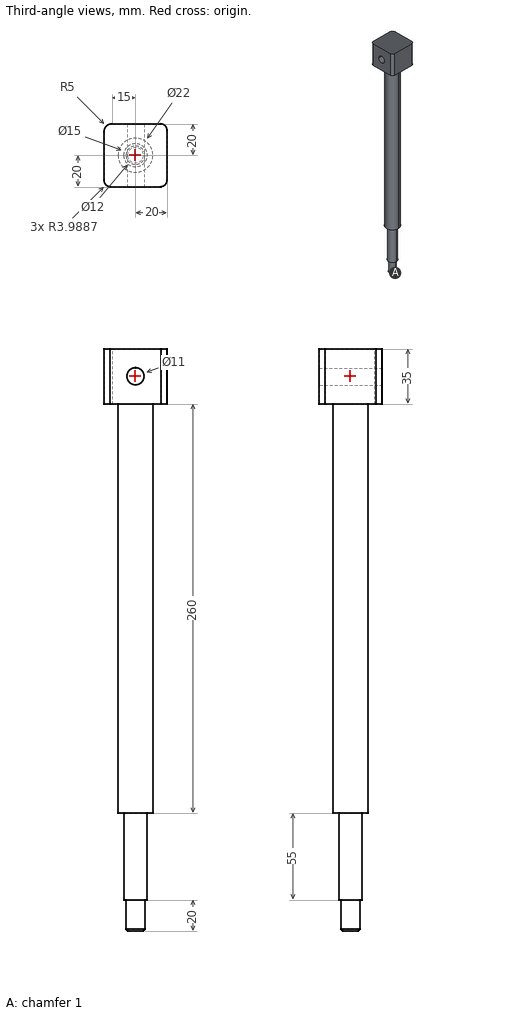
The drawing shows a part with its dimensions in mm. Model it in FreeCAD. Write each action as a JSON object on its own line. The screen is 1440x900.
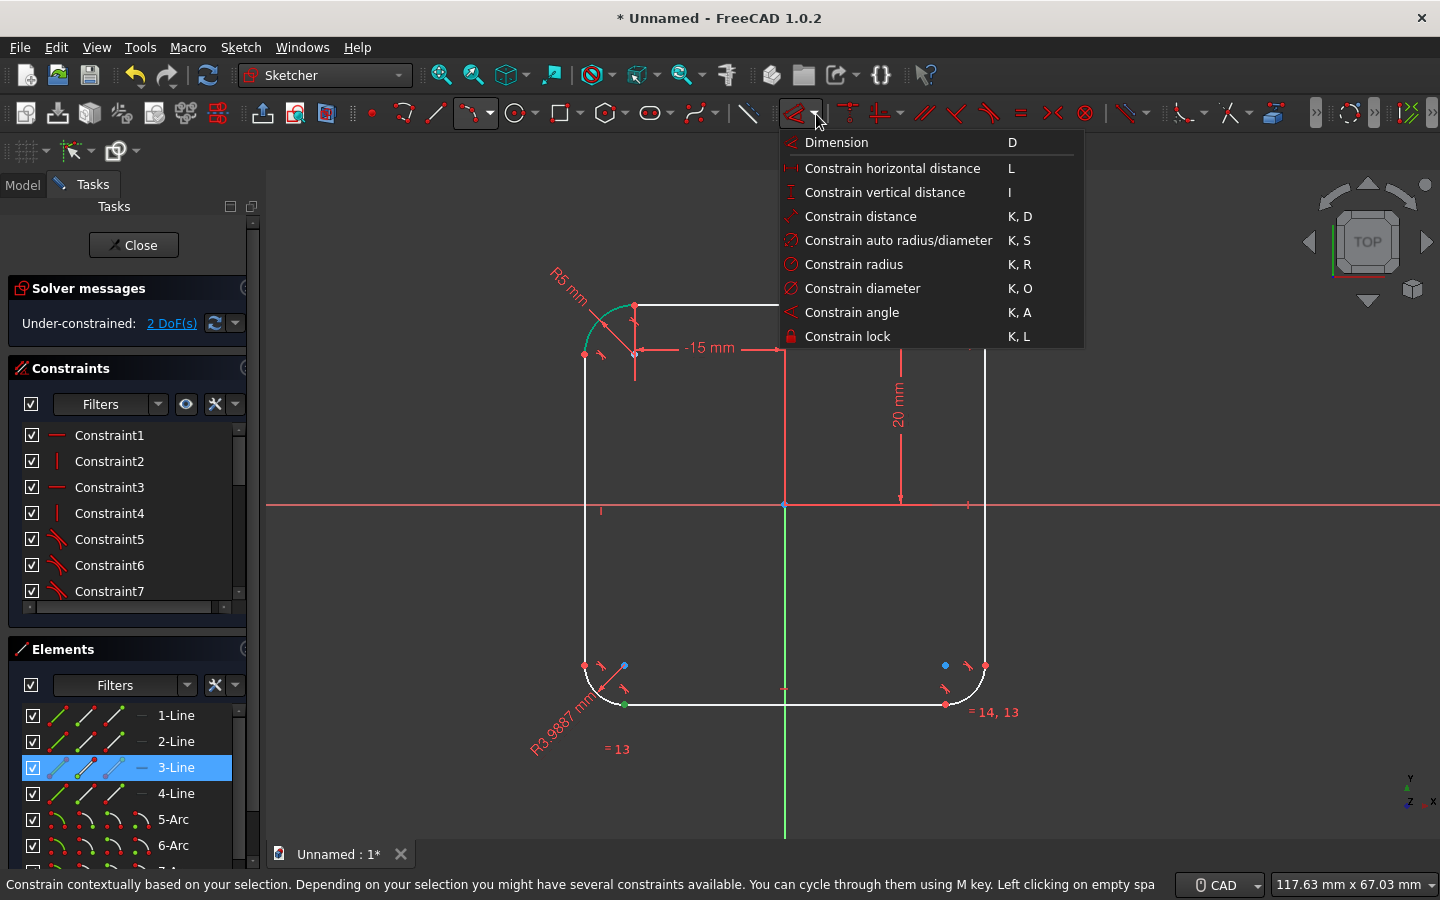
{"action": "left_click", "coordinate": [932, 192]}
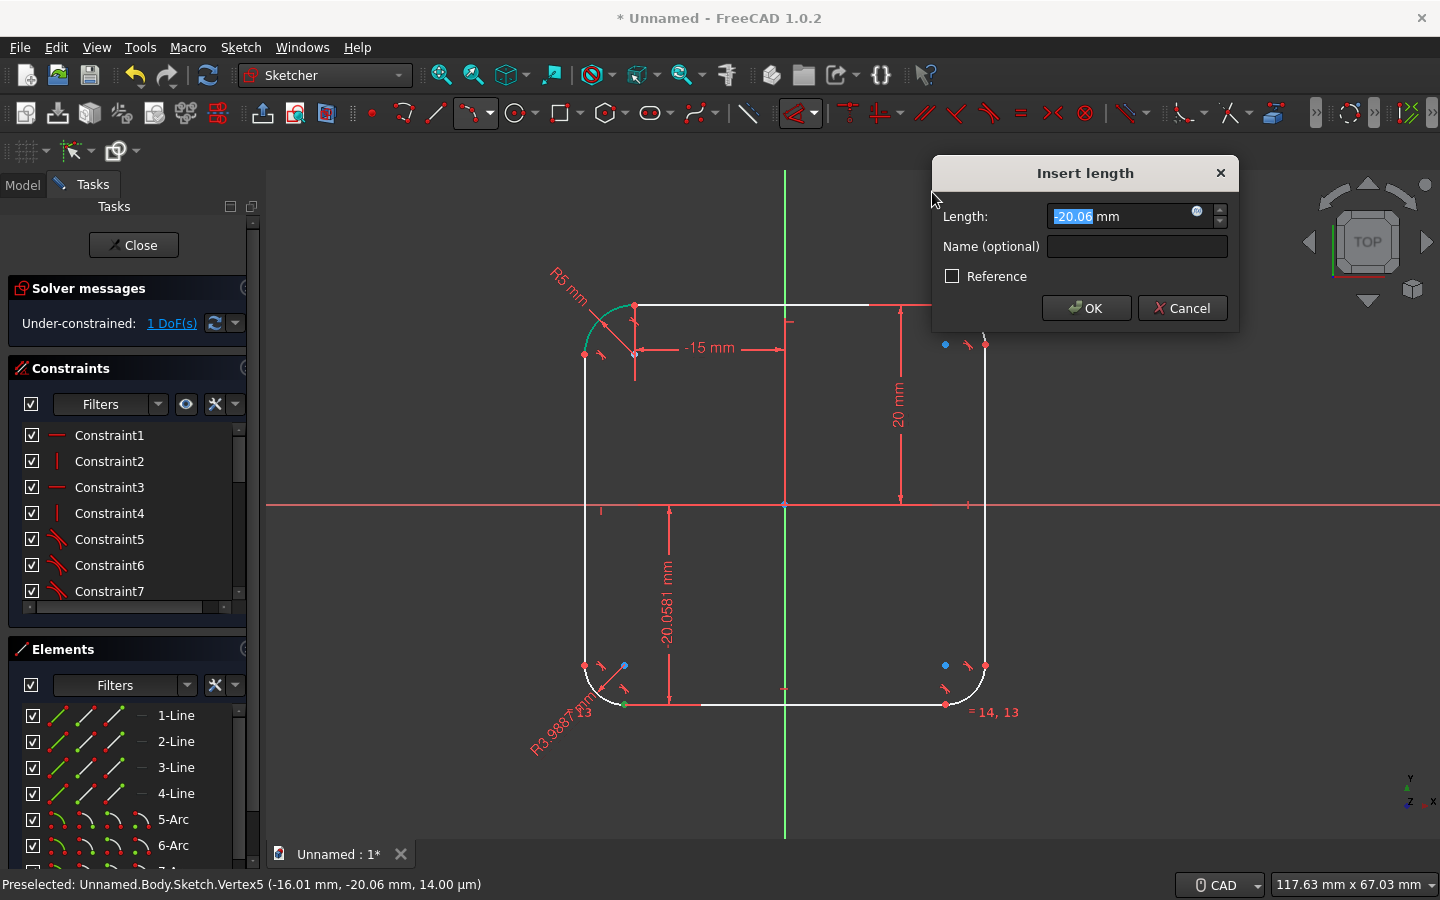
{"action": "type", "text": "-20"}
{"action": "key", "text": "Return"}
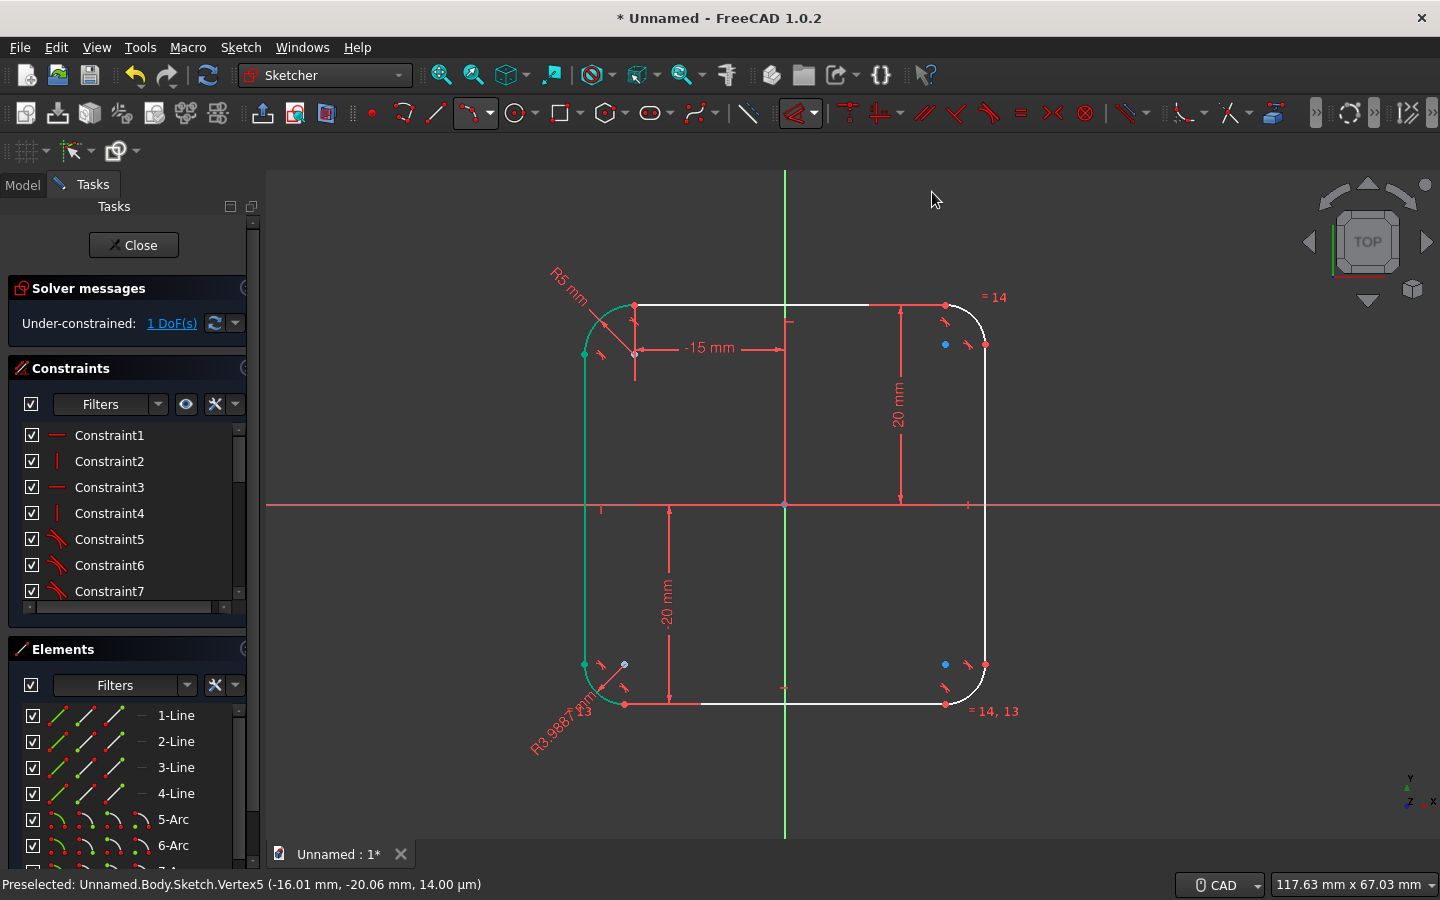
{"action": "left_click", "coordinate": [985, 664]}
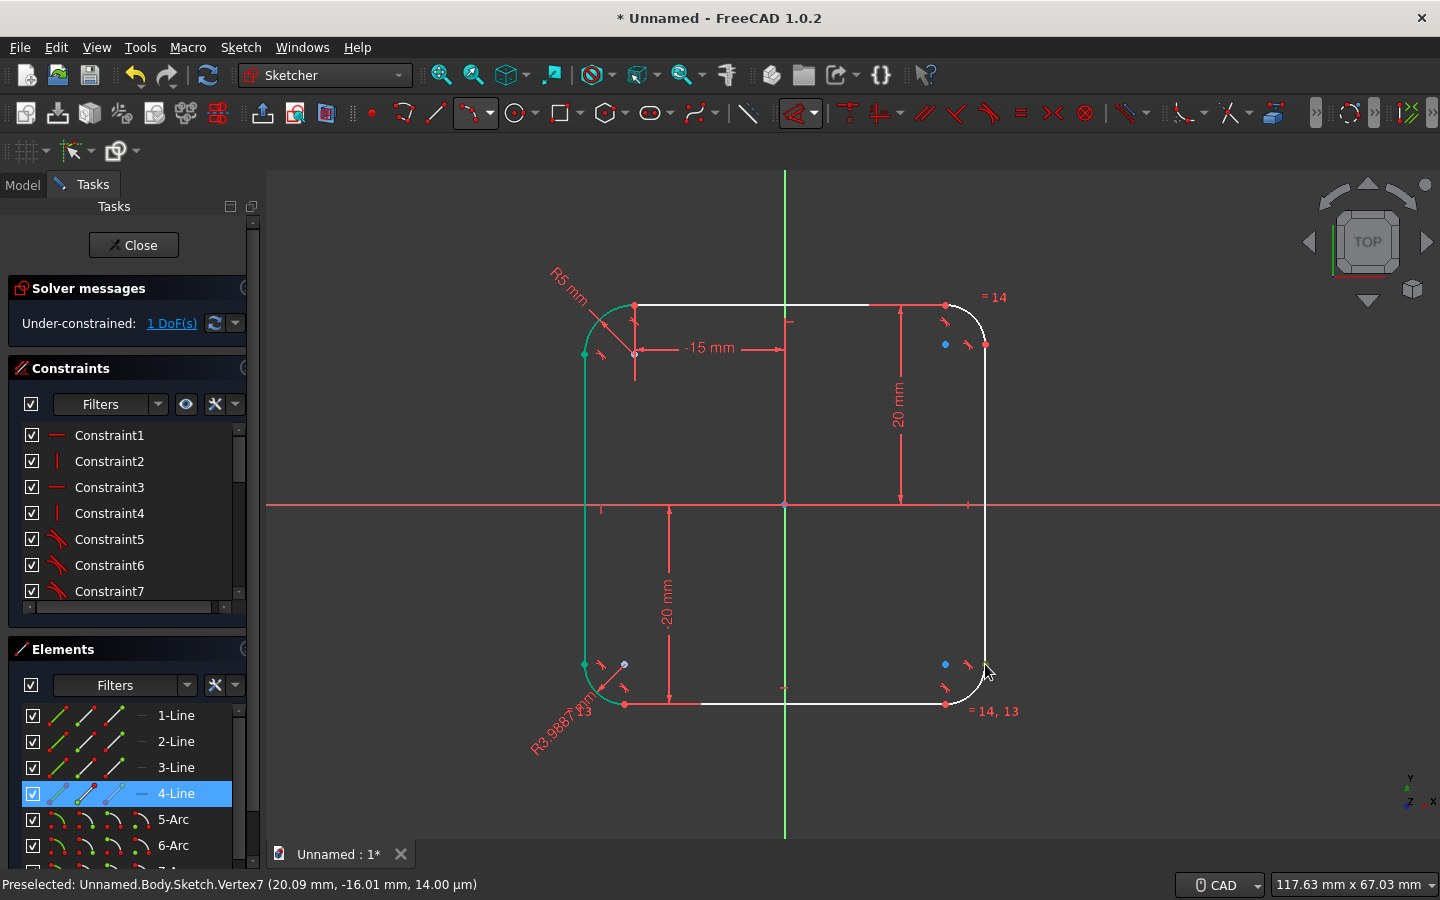
{"action": "left_click", "coordinate": [816, 114]}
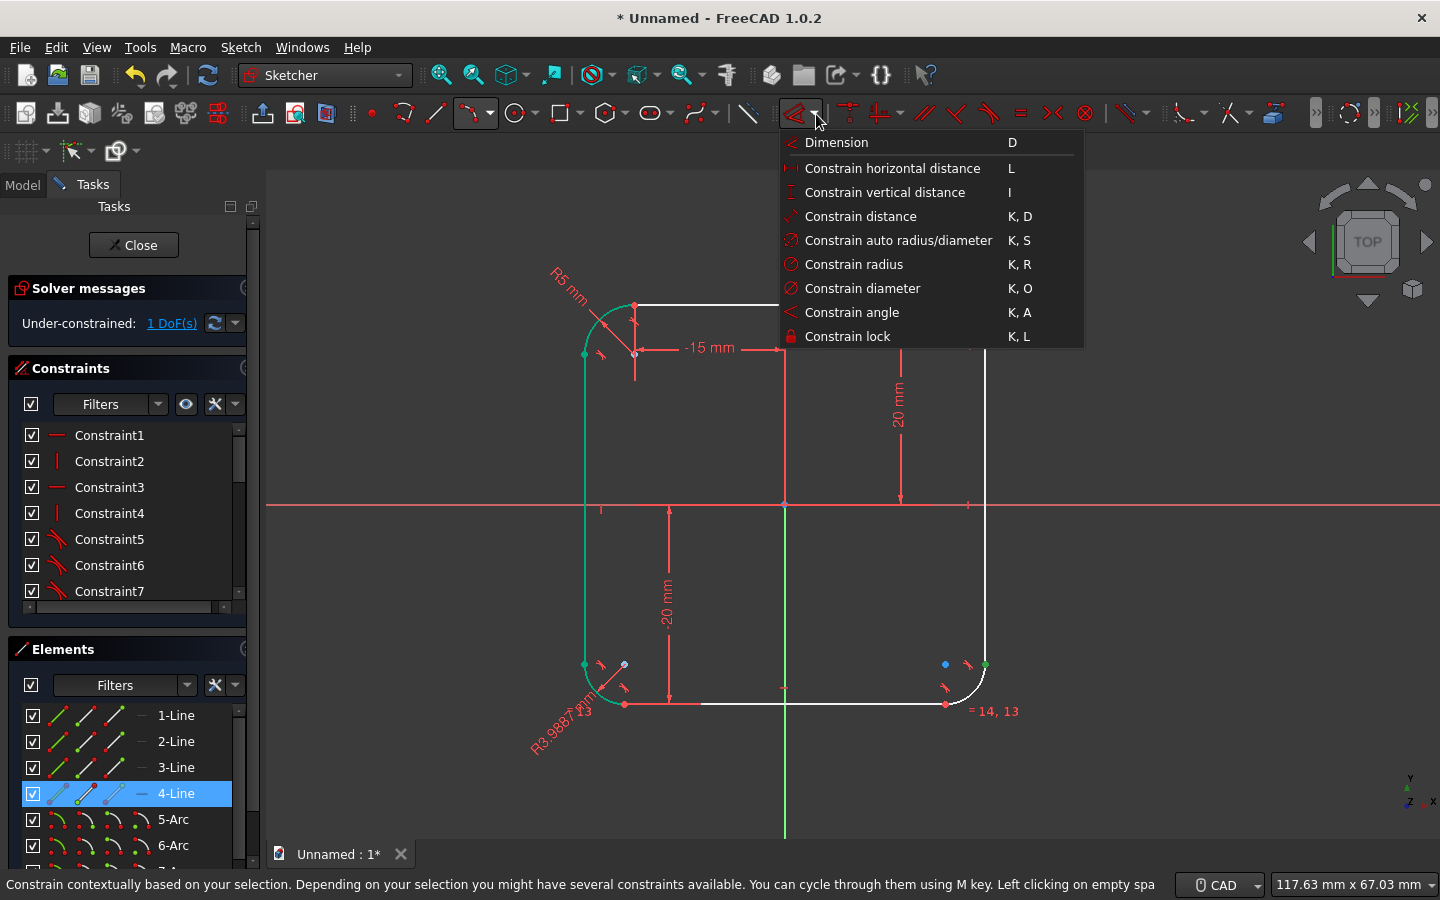
{"action": "left_click", "coordinate": [932, 168]}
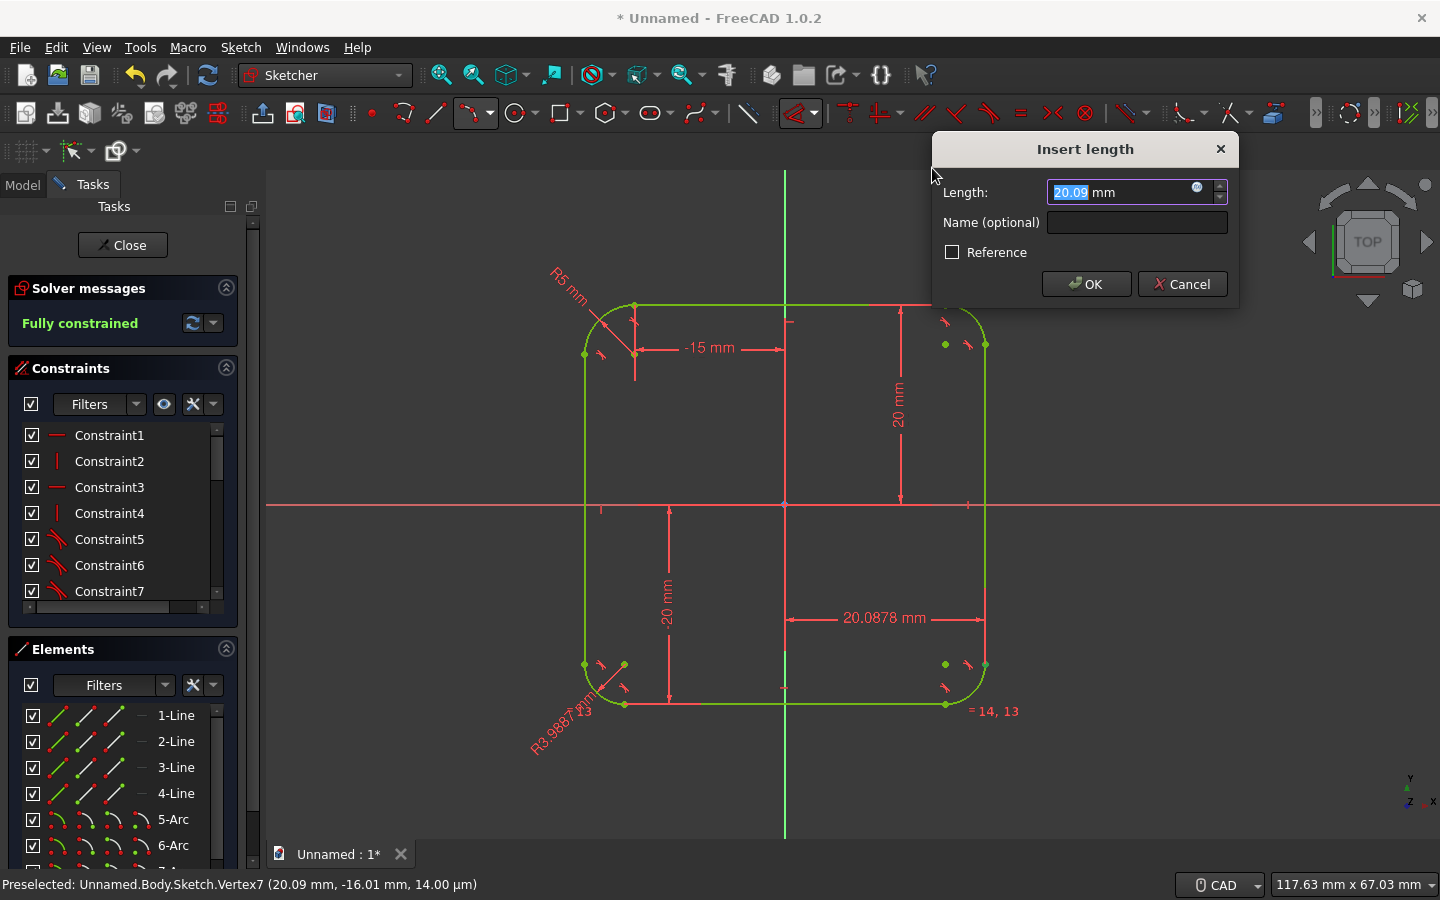
{"action": "type", "text": "20"}
{"action": "key", "text": "Return"}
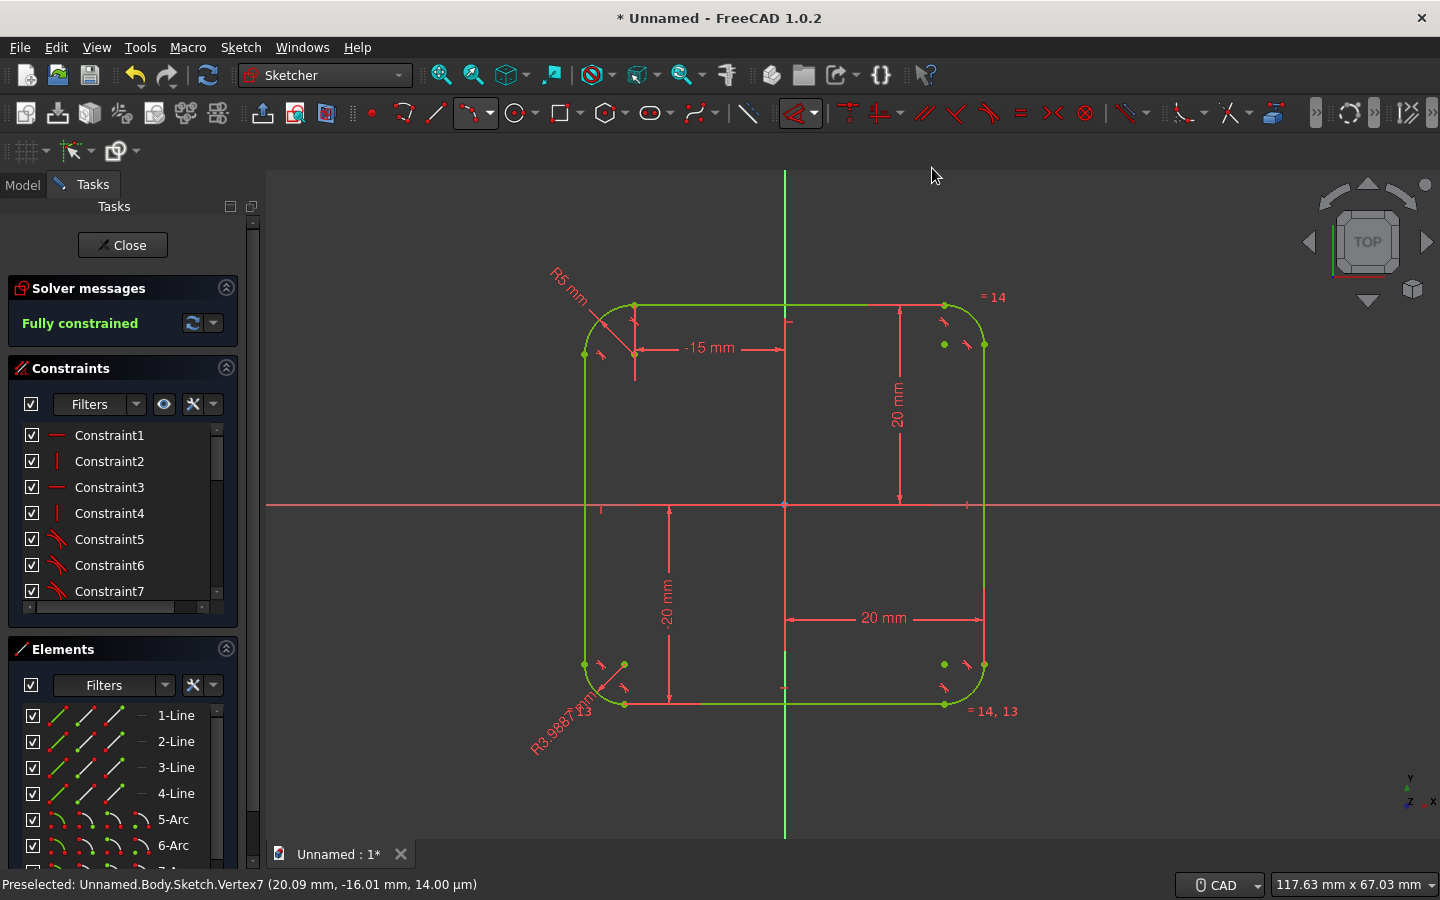
{"action": "left_click", "coordinate": [123, 245]}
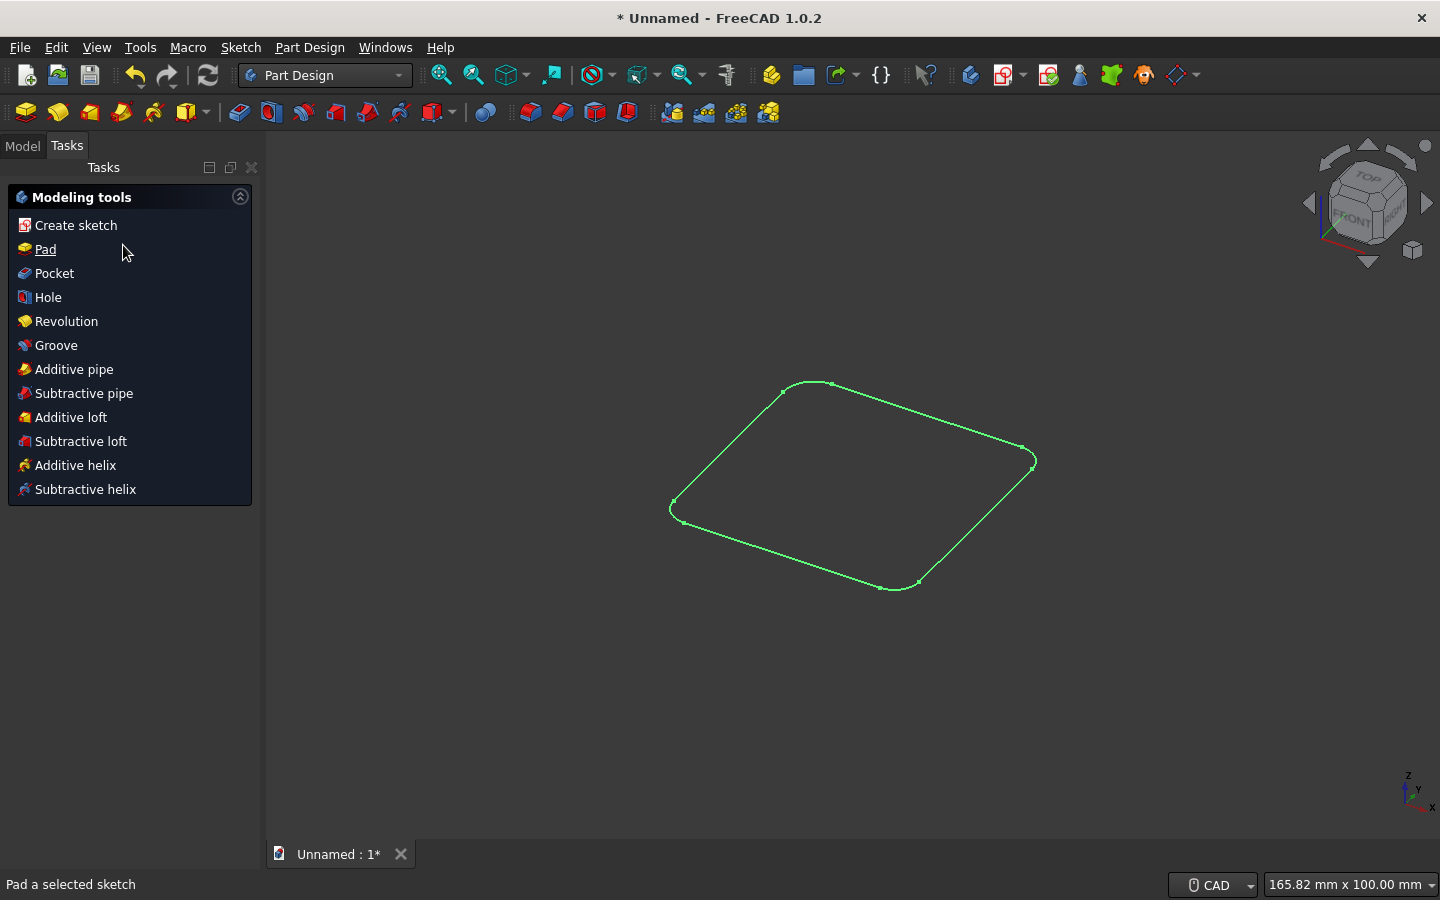
{"action": "left_click", "coordinate": [26, 112]}